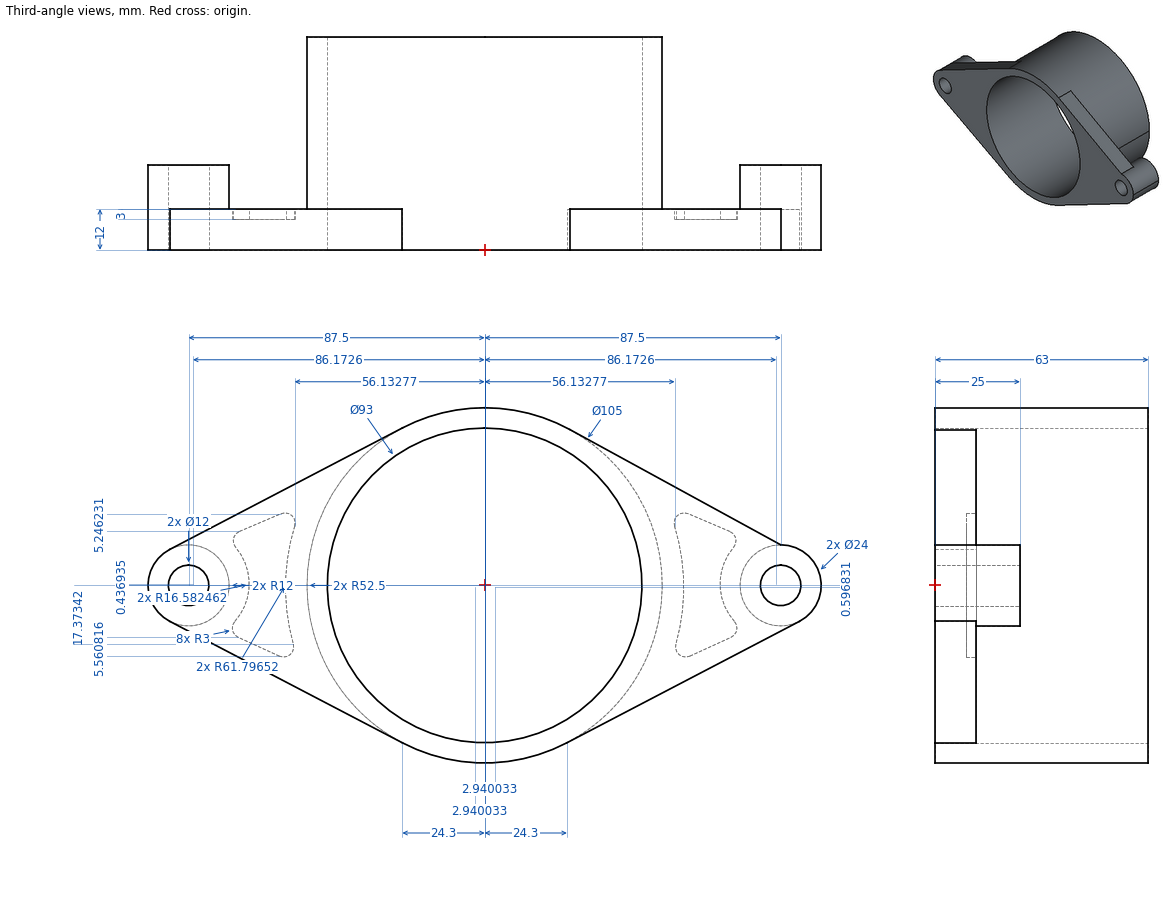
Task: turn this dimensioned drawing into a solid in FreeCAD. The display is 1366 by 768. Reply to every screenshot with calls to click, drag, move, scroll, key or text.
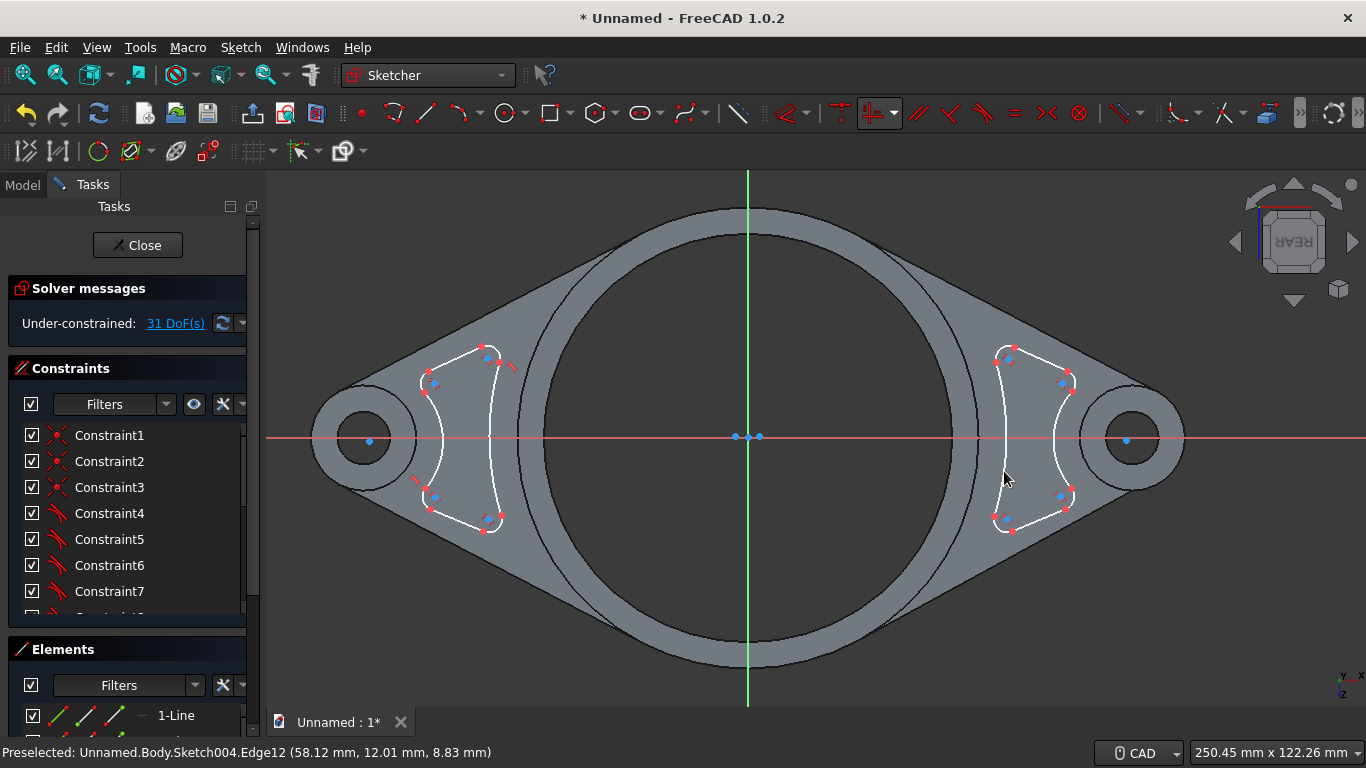
click(1004, 471)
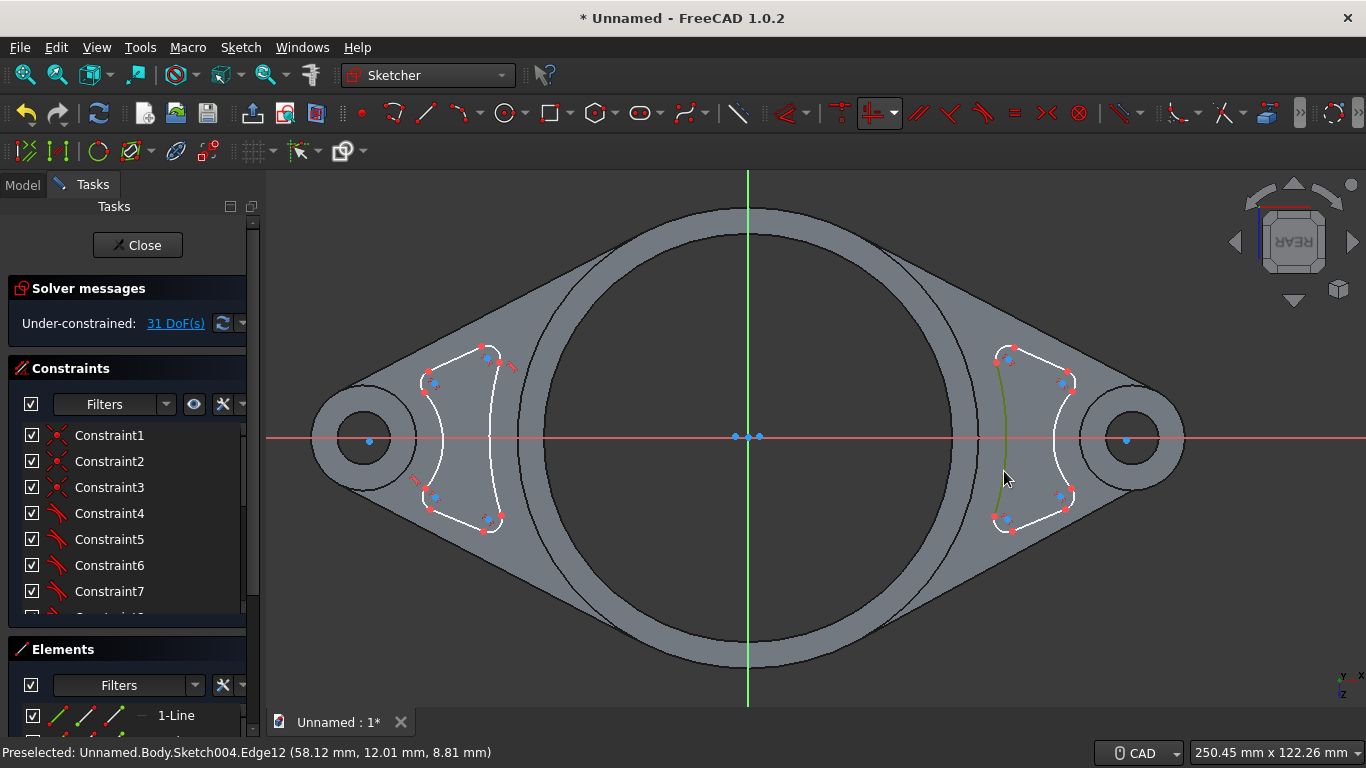
click(999, 529)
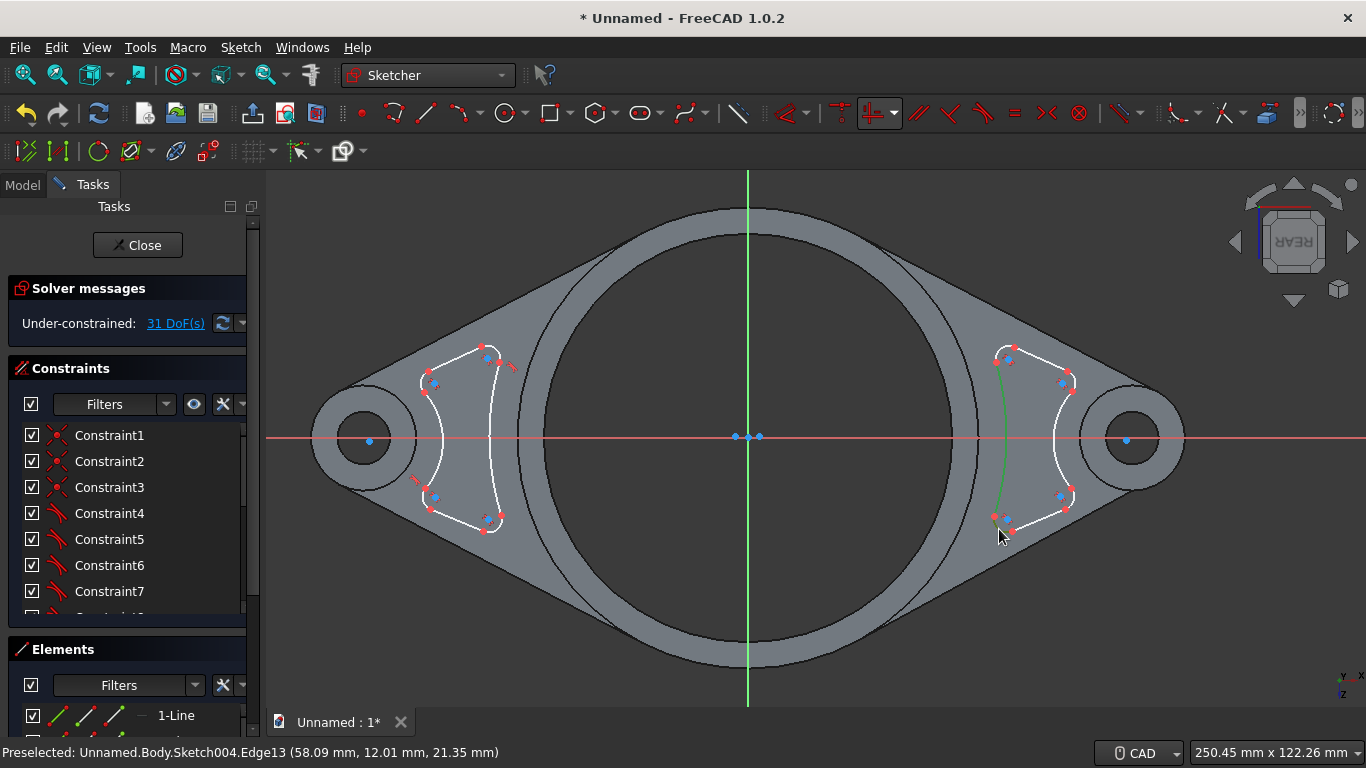
click(984, 114)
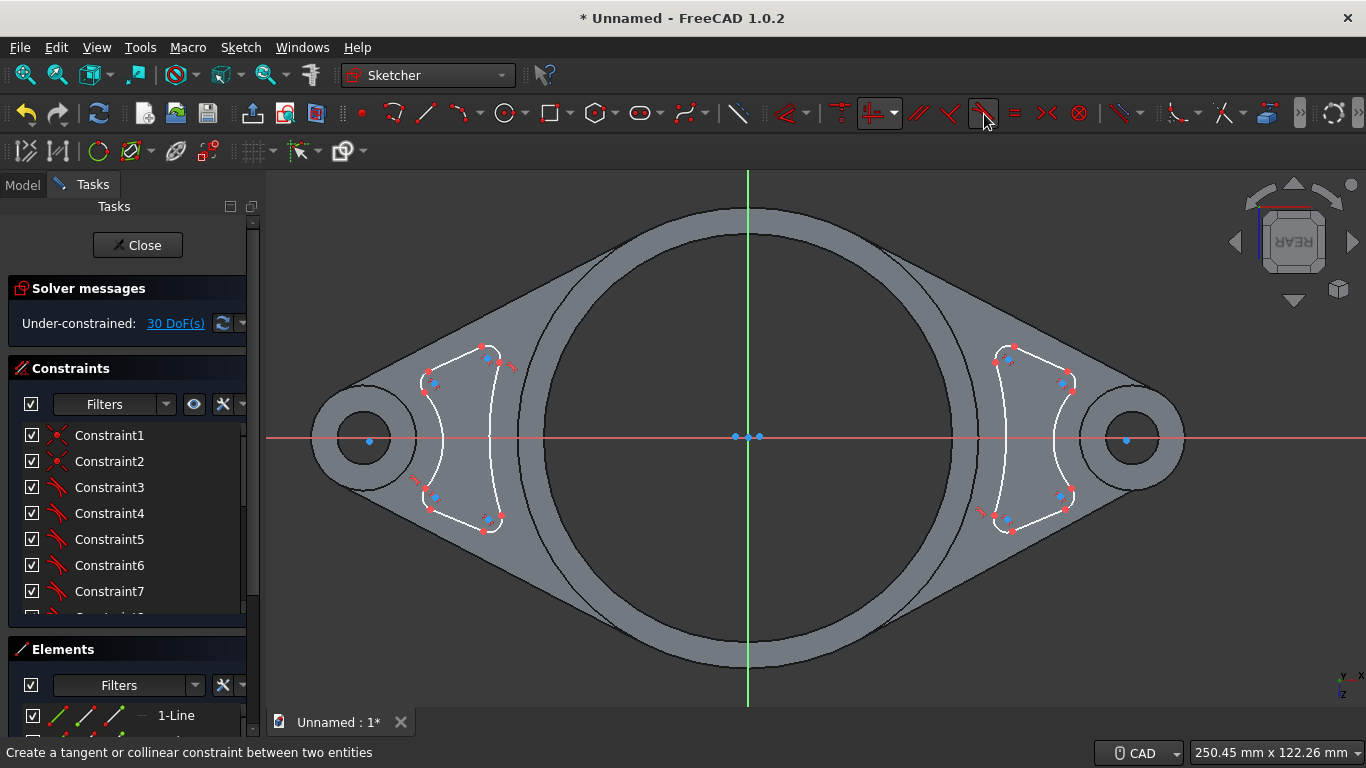
click(1074, 500)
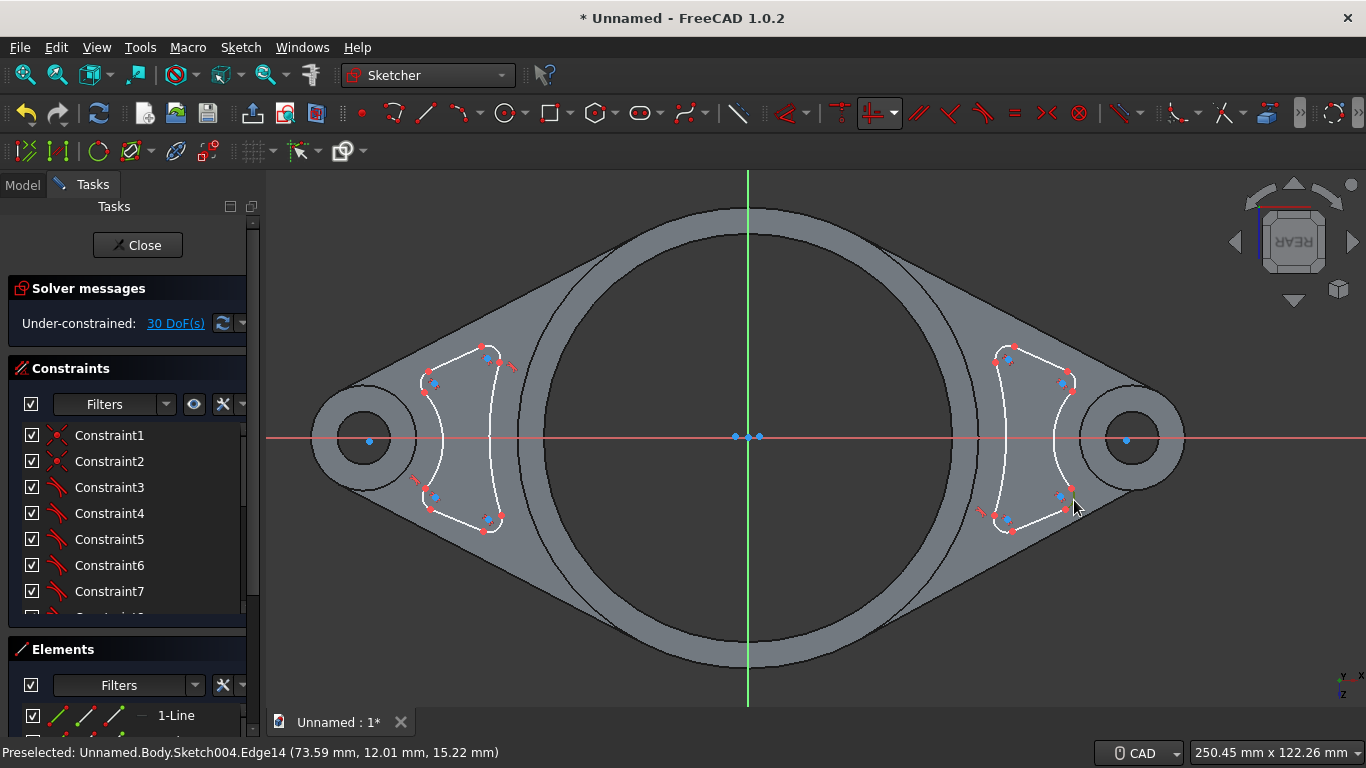
click(1057, 419)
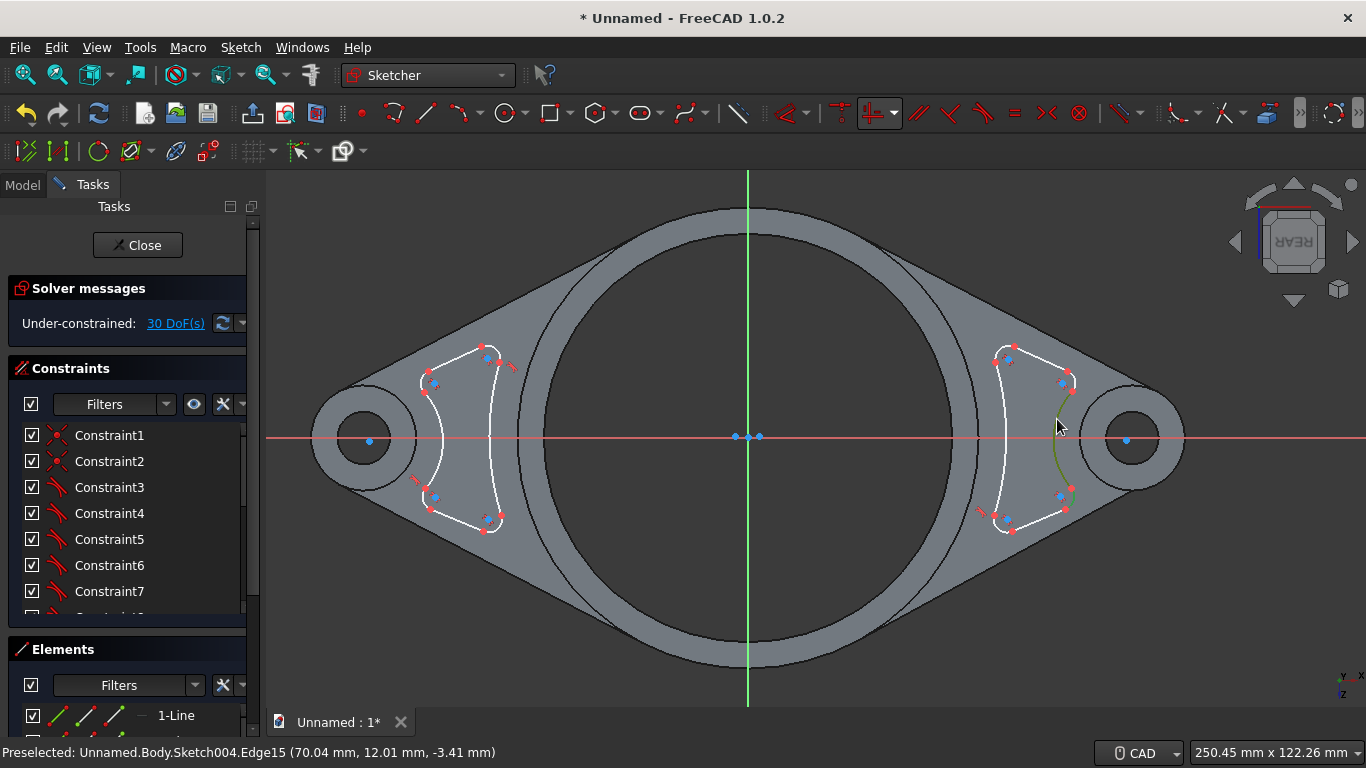
click(984, 114)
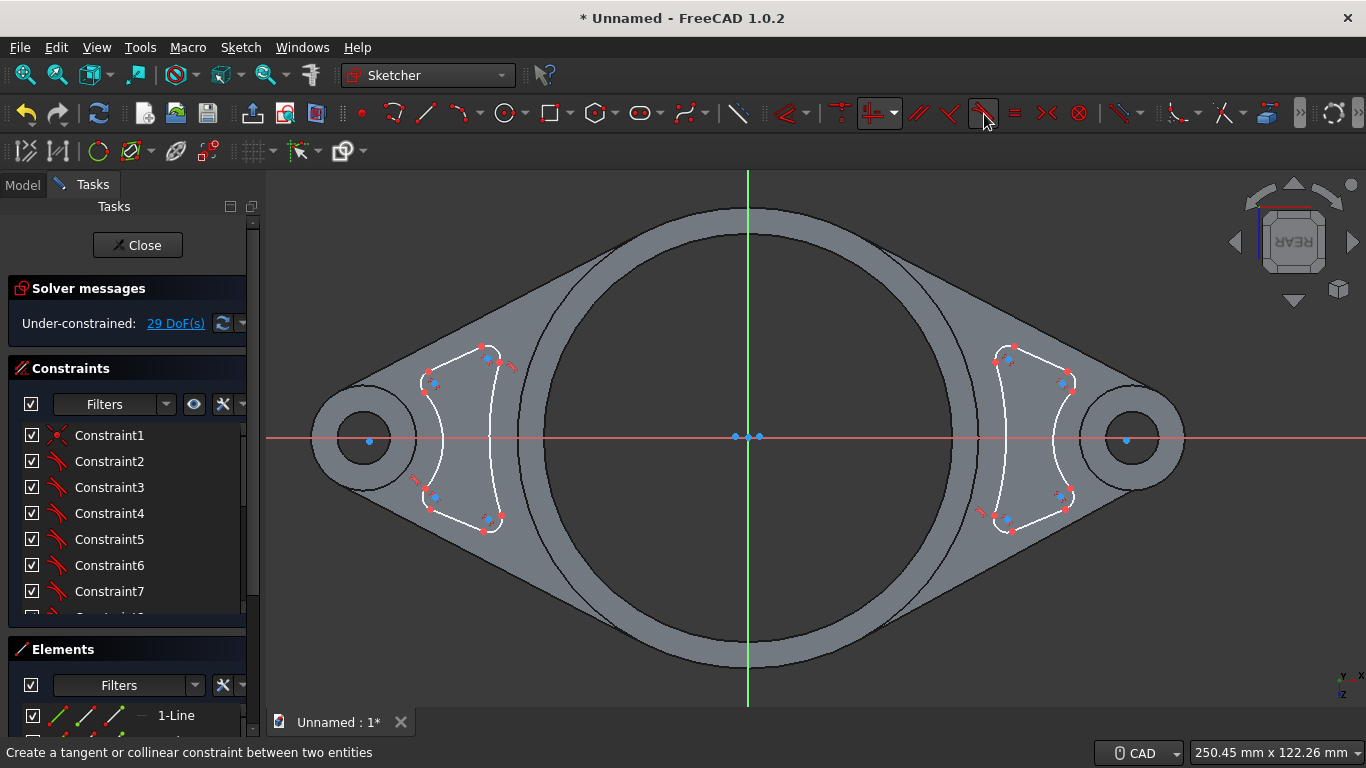
click(1057, 419)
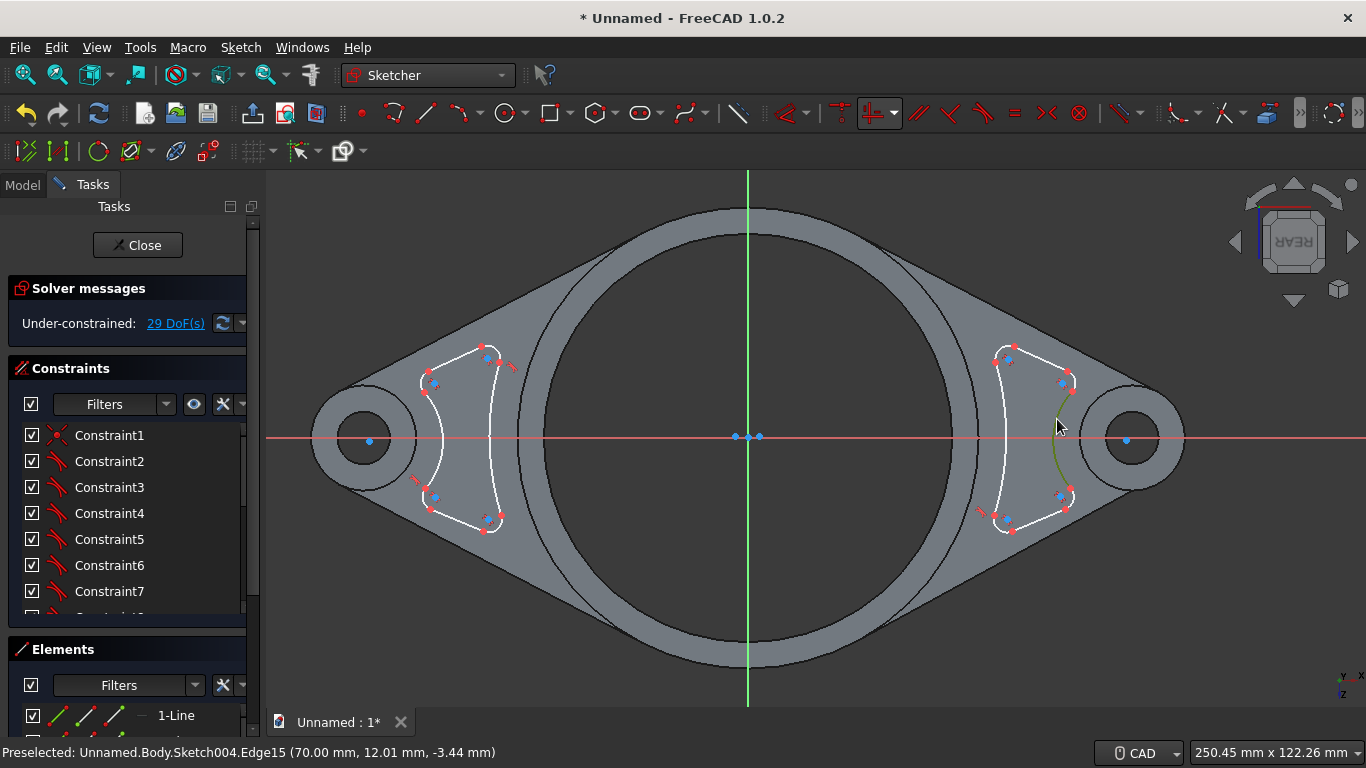
click(1075, 380)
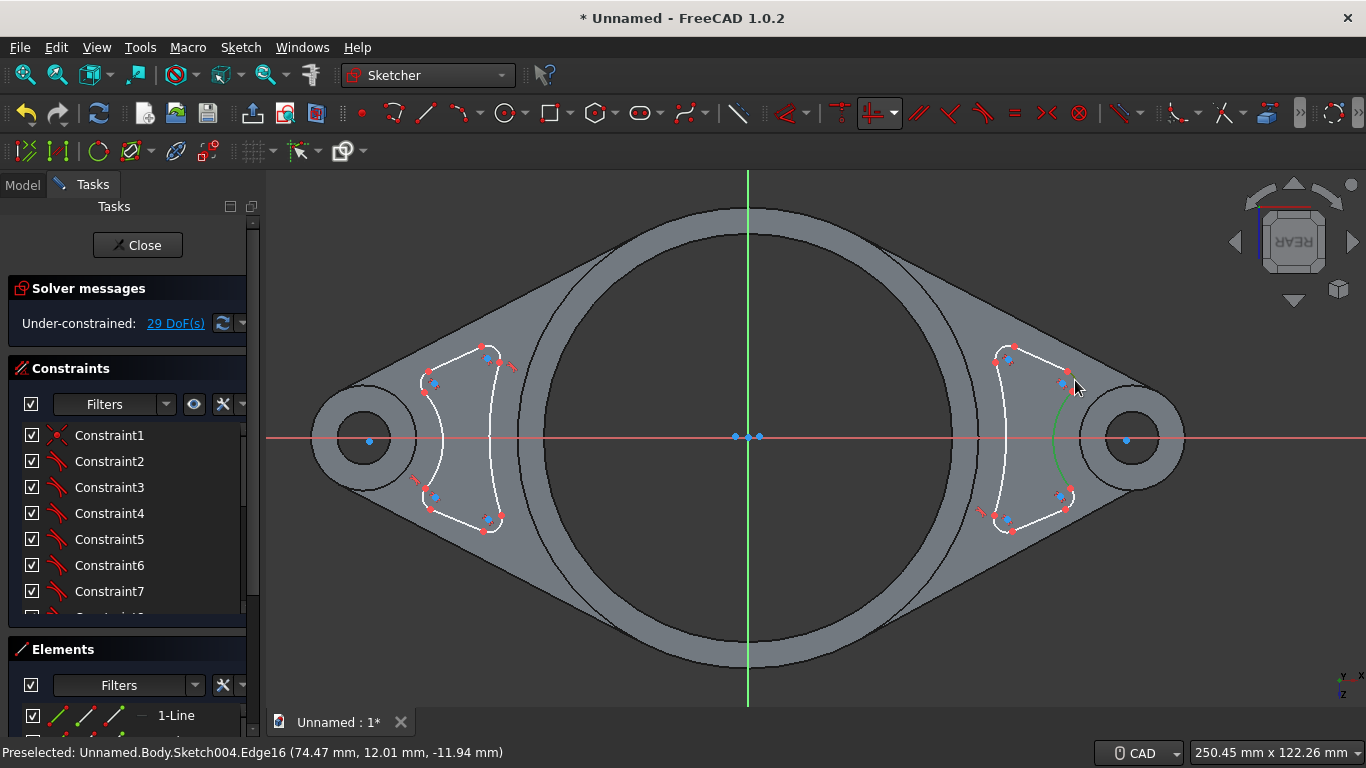
key(t)